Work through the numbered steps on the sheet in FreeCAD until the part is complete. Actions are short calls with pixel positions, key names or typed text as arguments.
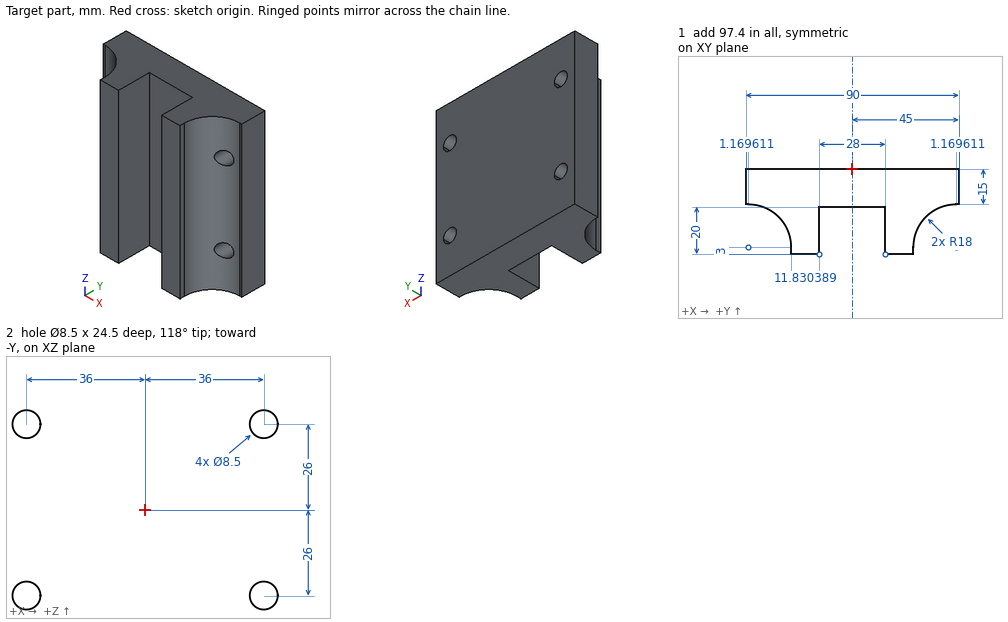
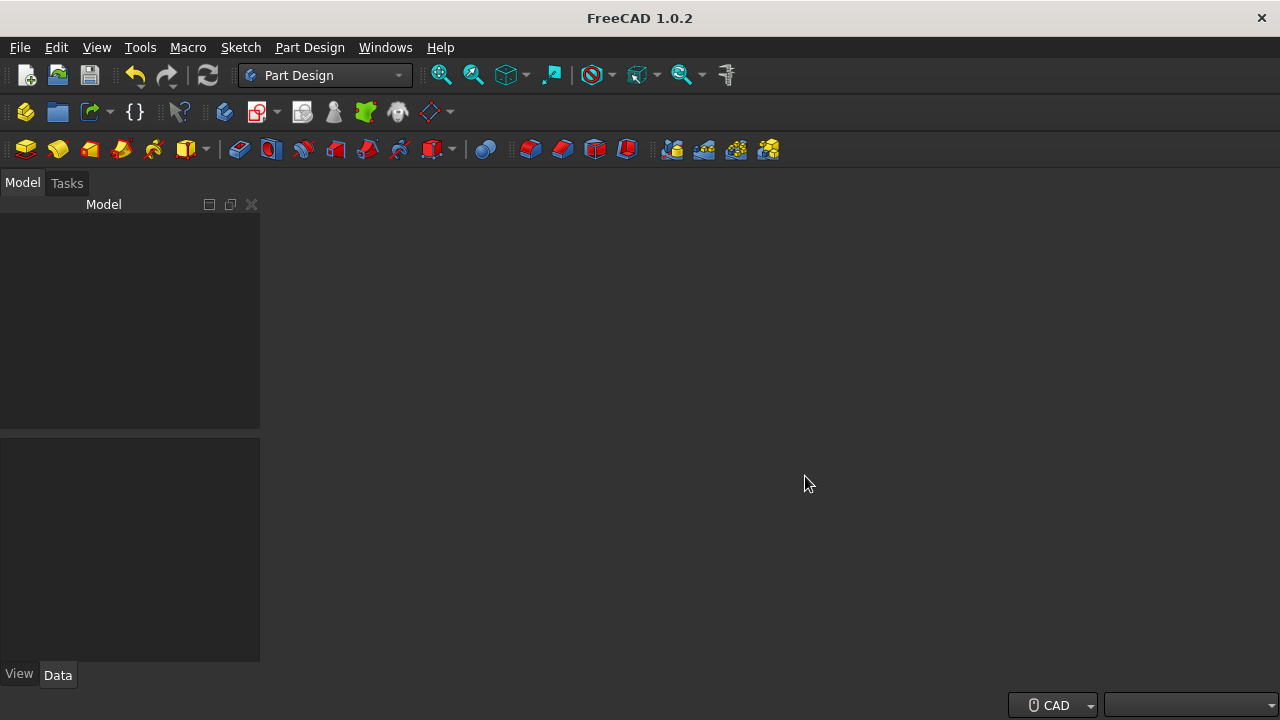
click(26, 76)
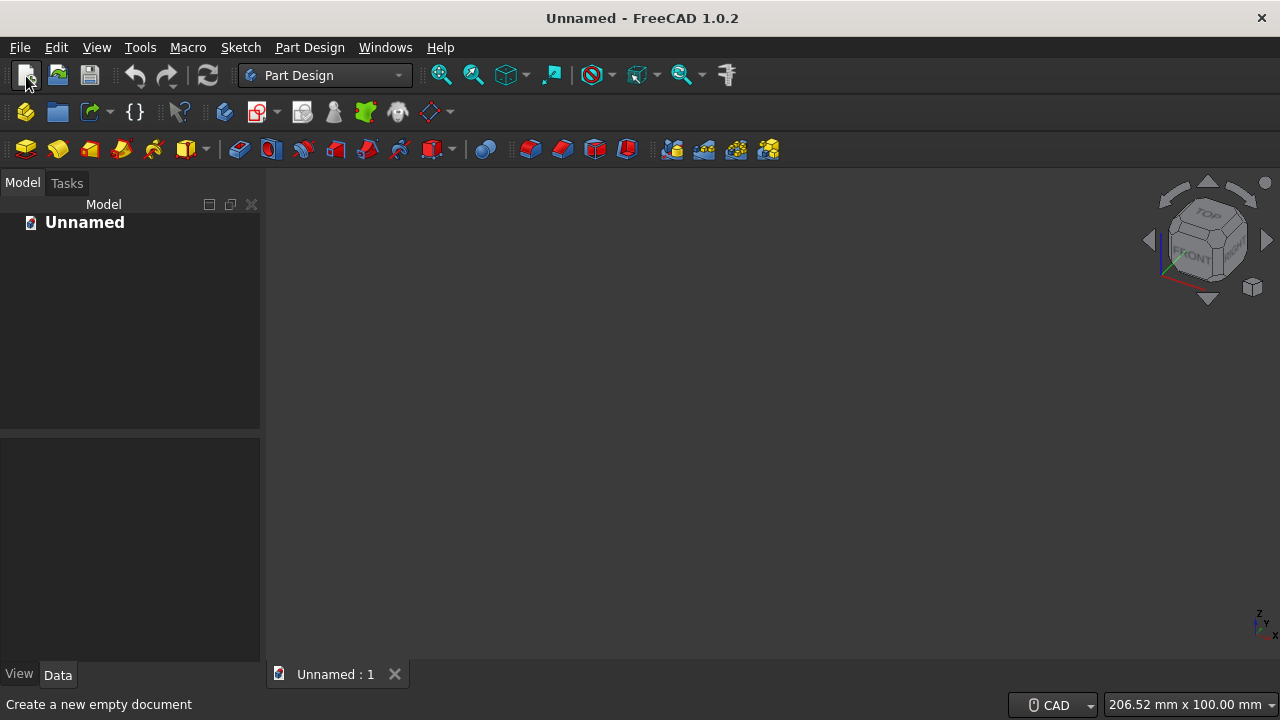
click(258, 112)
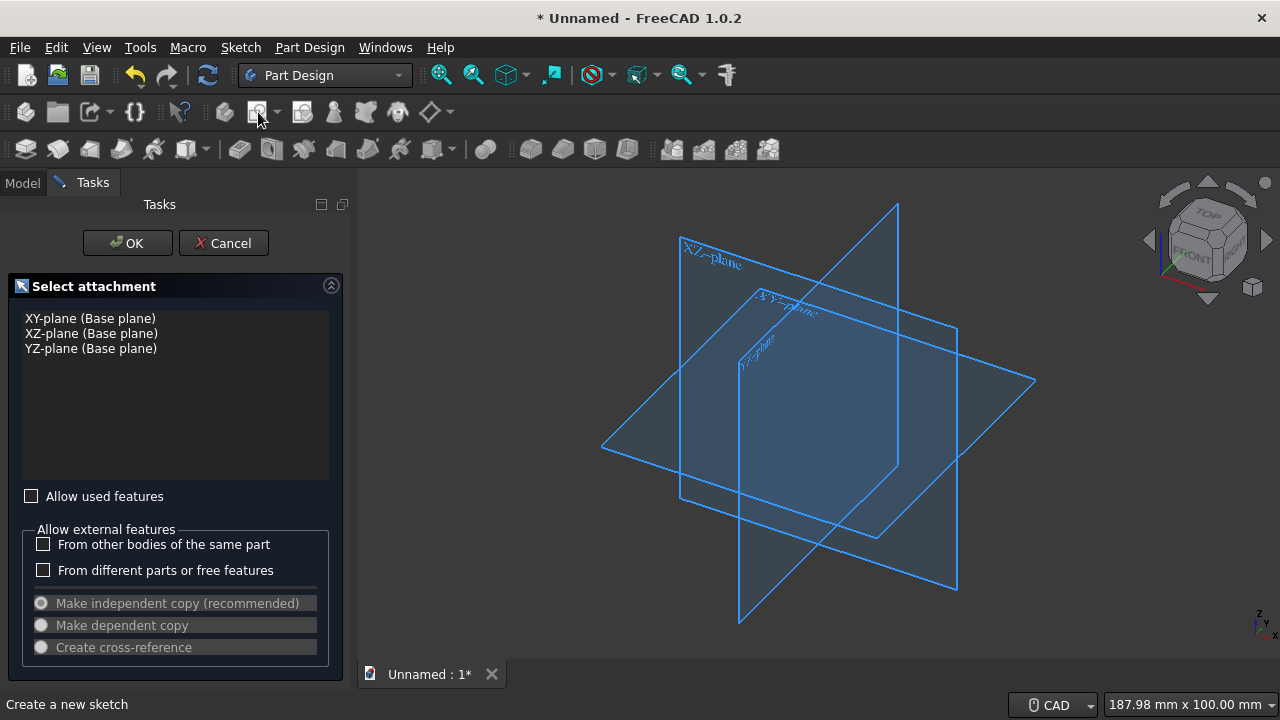
click(82, 318)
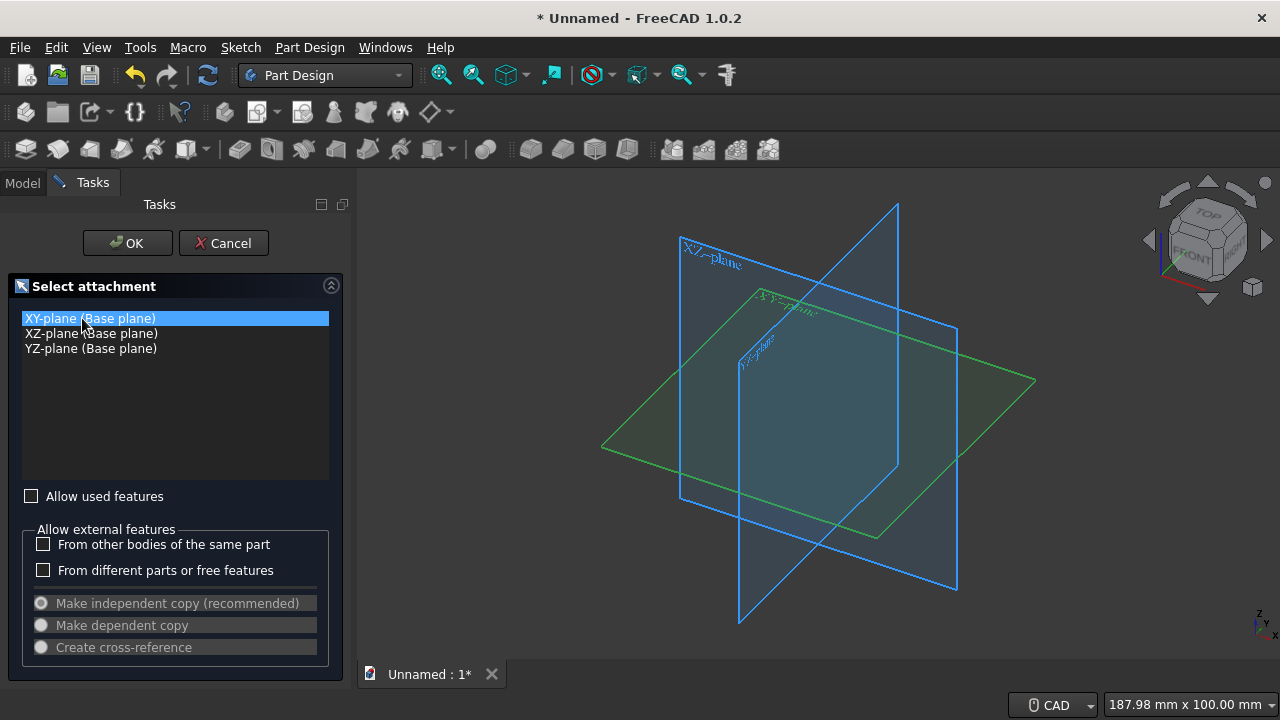
click(128, 243)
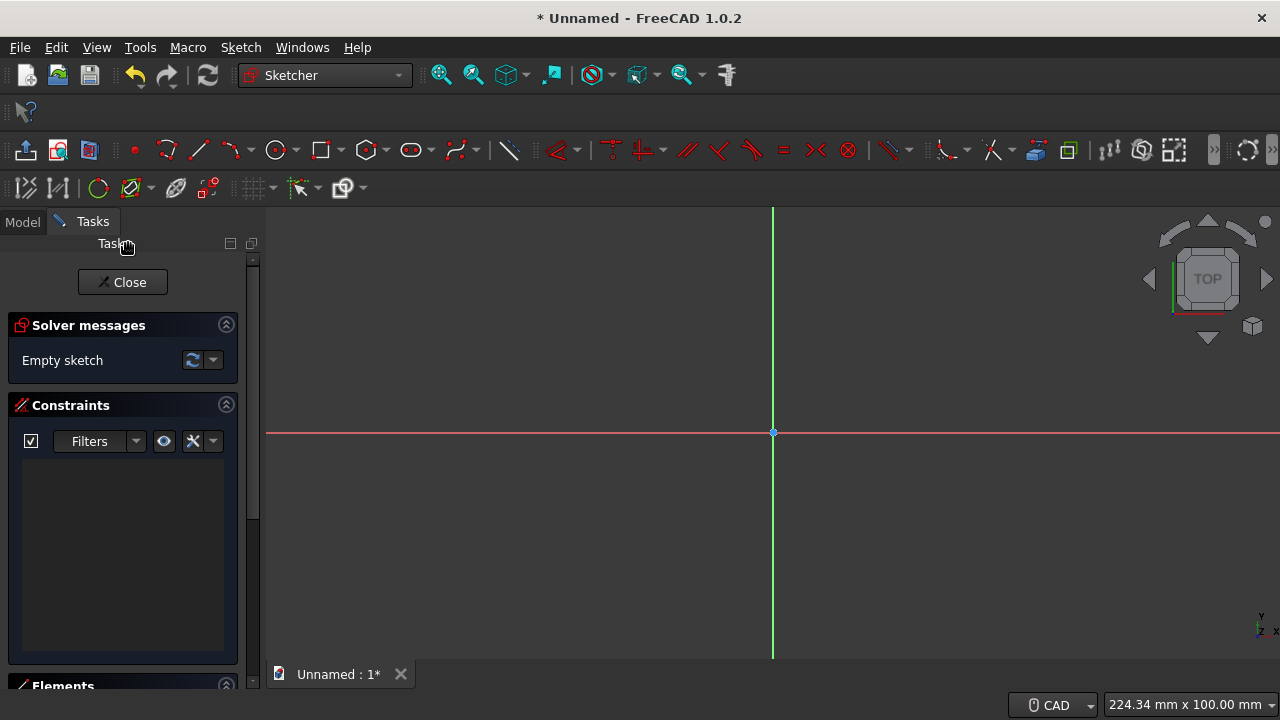
scroll(912, 631, up, 2)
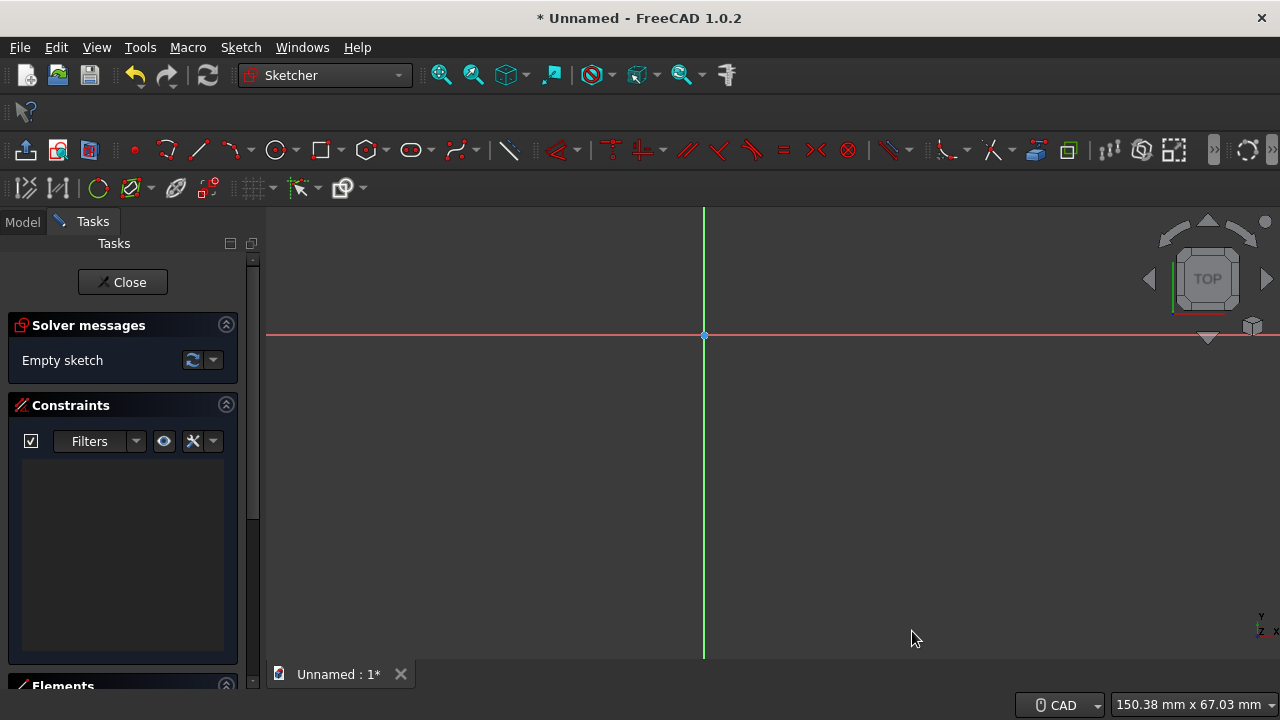
key(g)
key(m)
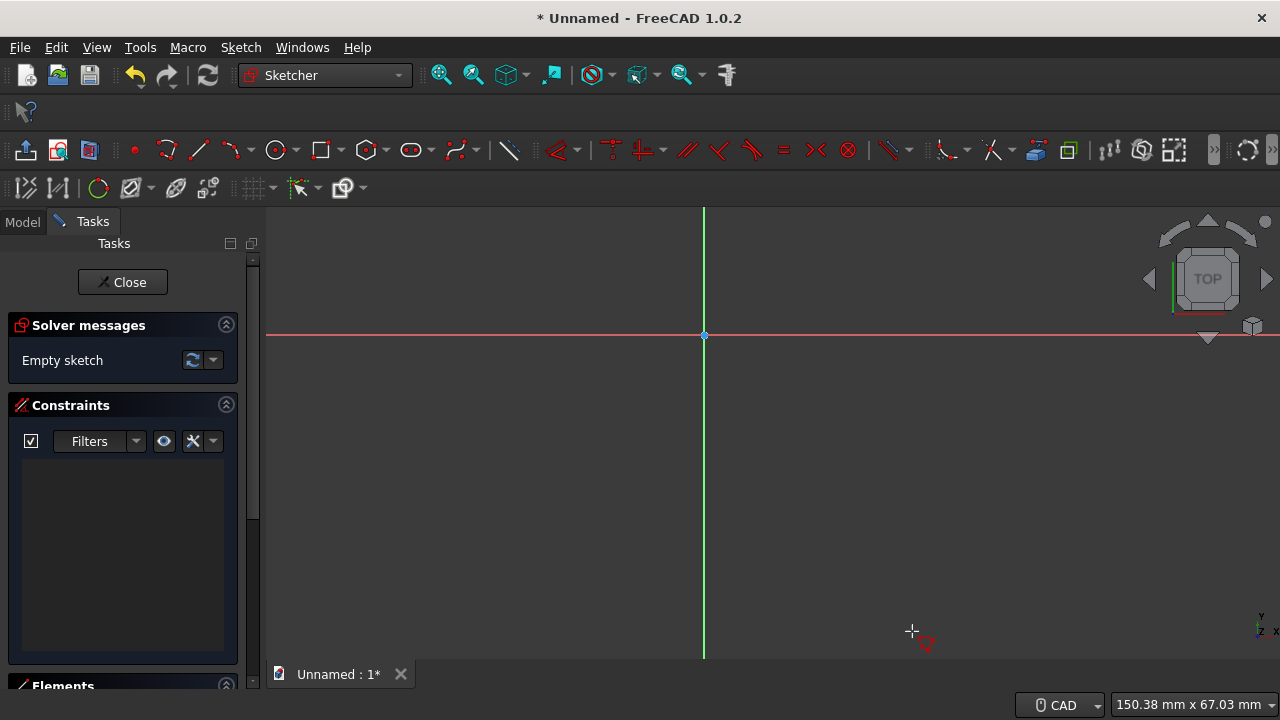
click(530, 558)
click(530, 578)
click(610, 578)
click(610, 443)
click(799, 443)
click(799, 578)
click(878, 578)
click(878, 558)
right_click(878, 558)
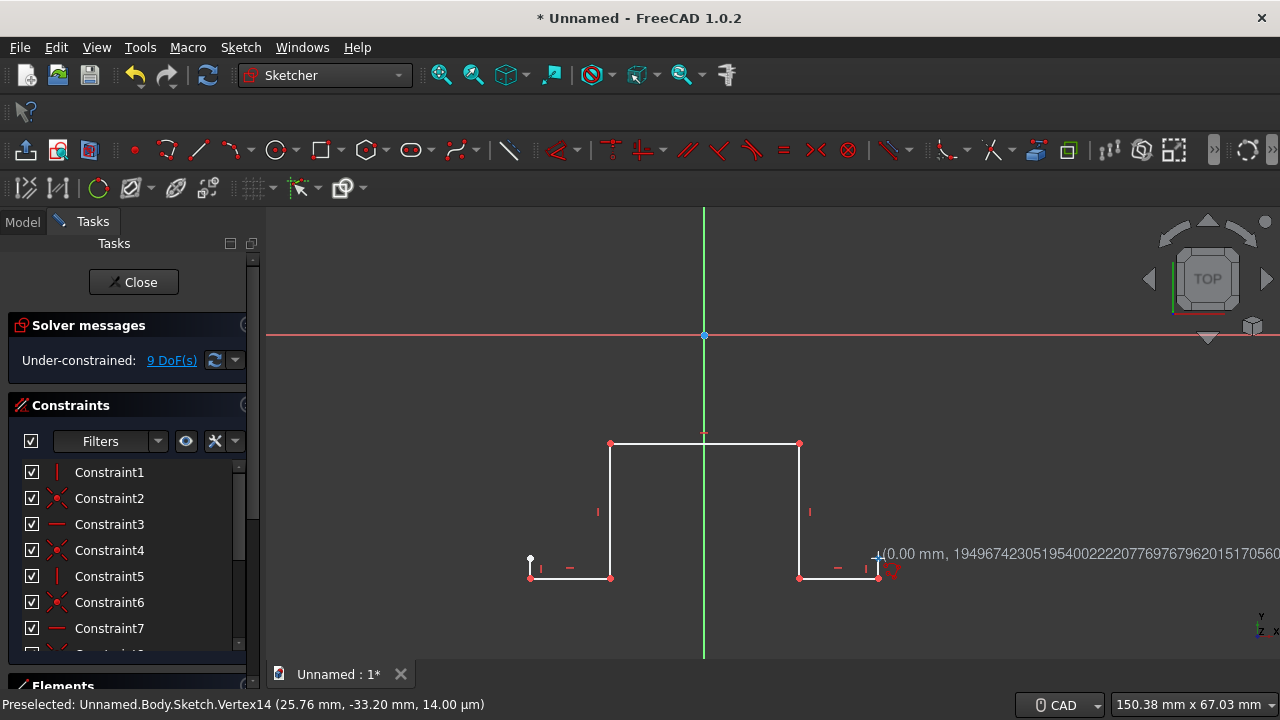
click(1000, 436)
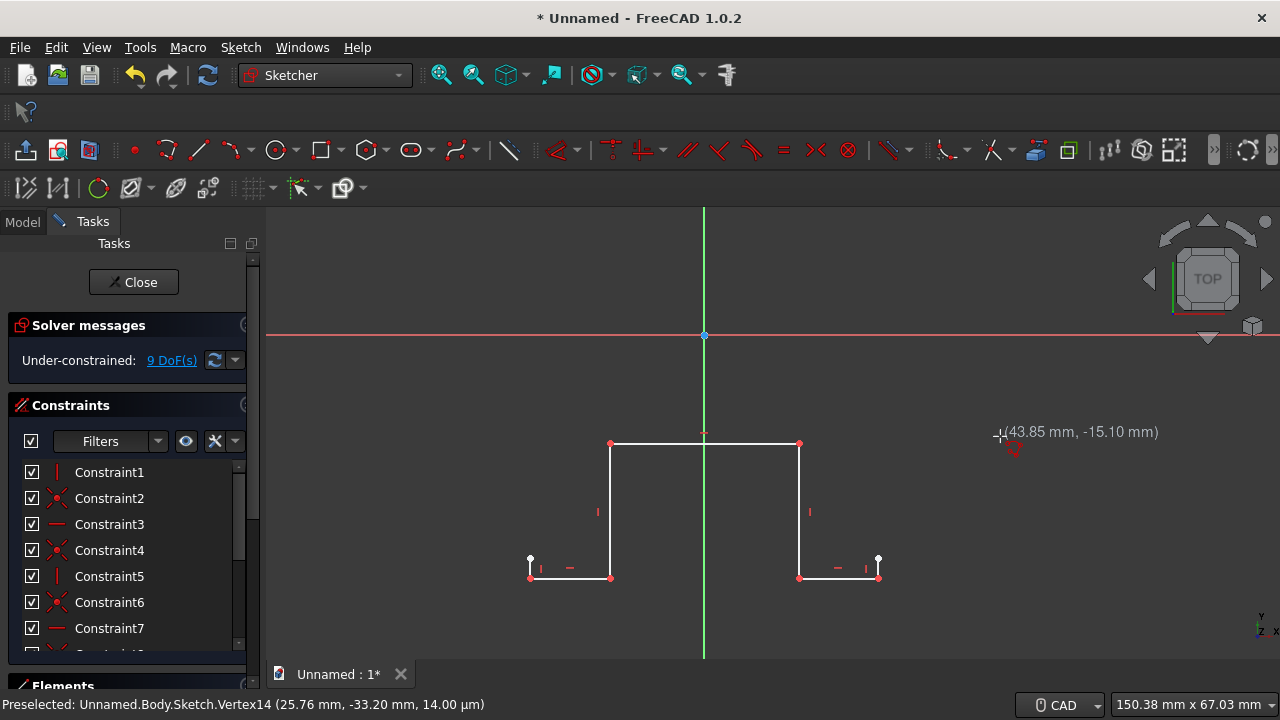
scroll(1008, 436, up, 4)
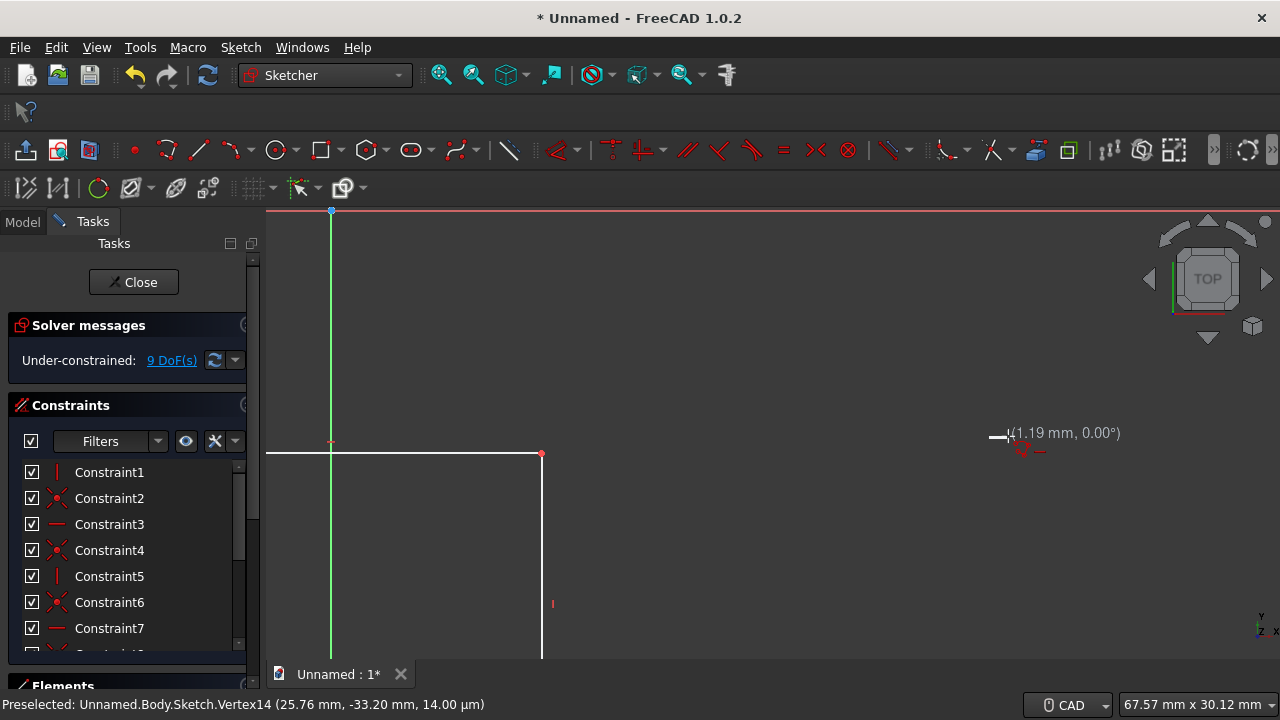
click(1007, 435)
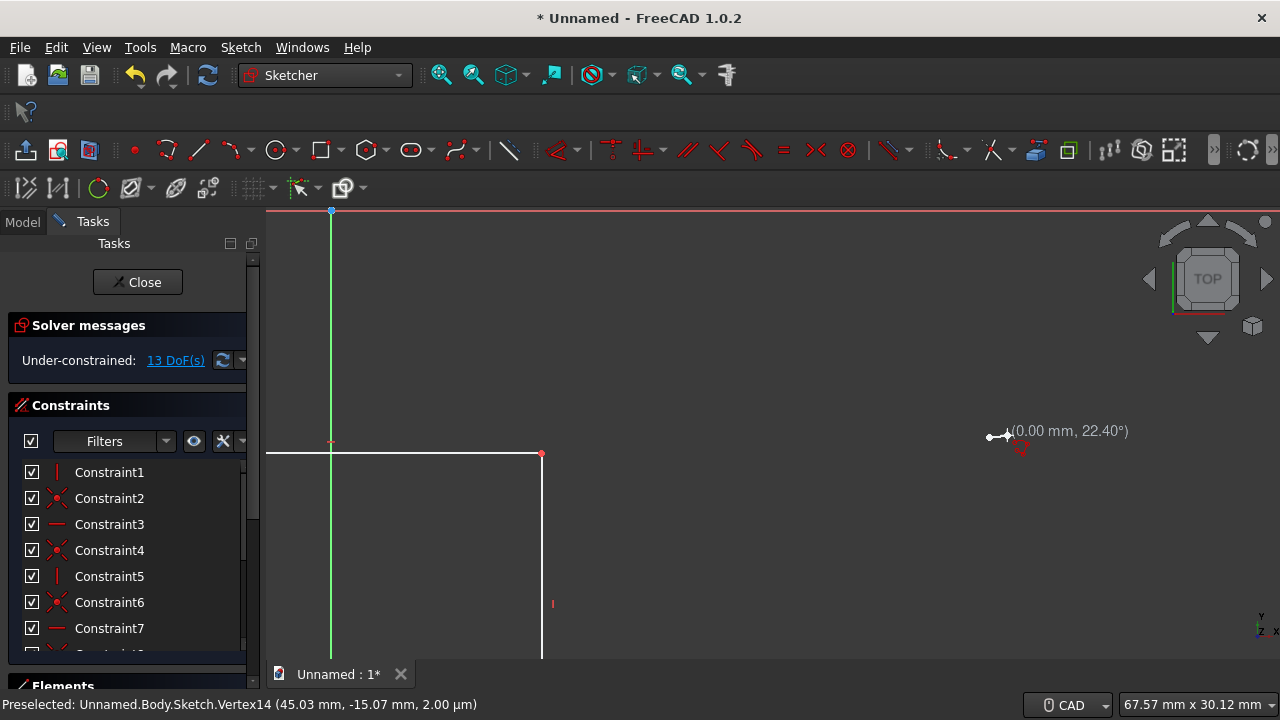
scroll(1009, 394, down, 4)